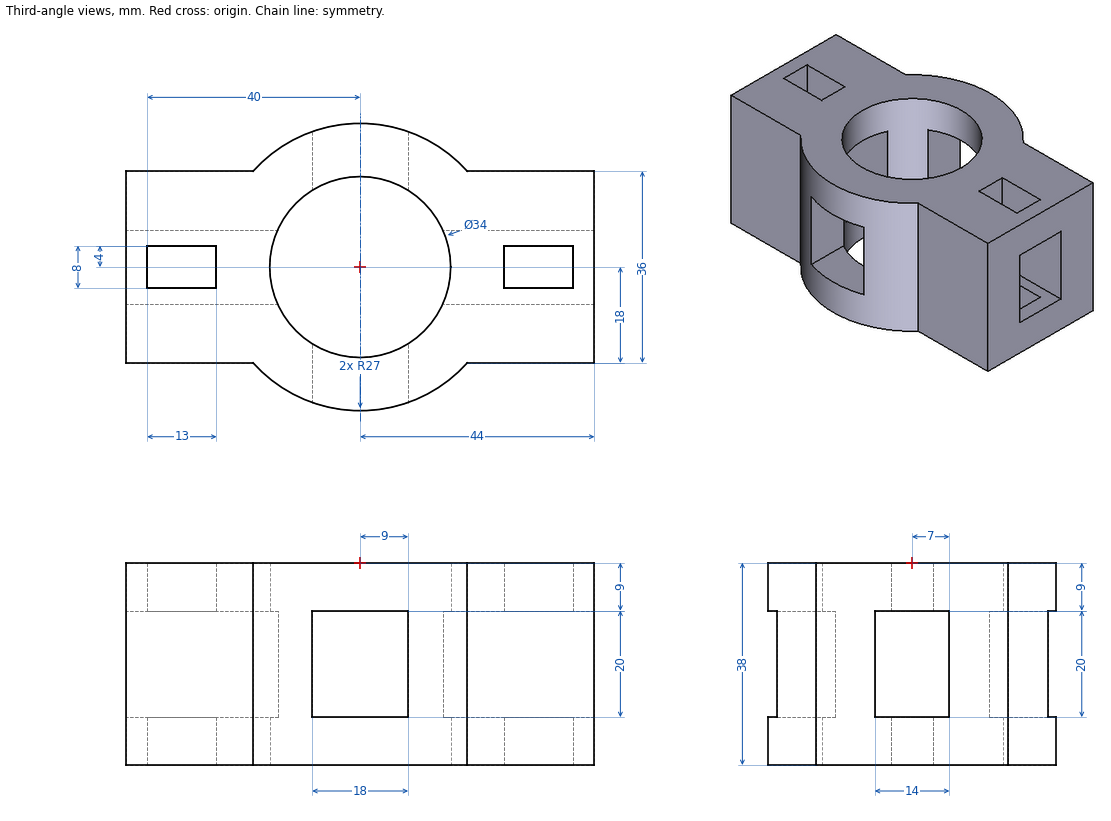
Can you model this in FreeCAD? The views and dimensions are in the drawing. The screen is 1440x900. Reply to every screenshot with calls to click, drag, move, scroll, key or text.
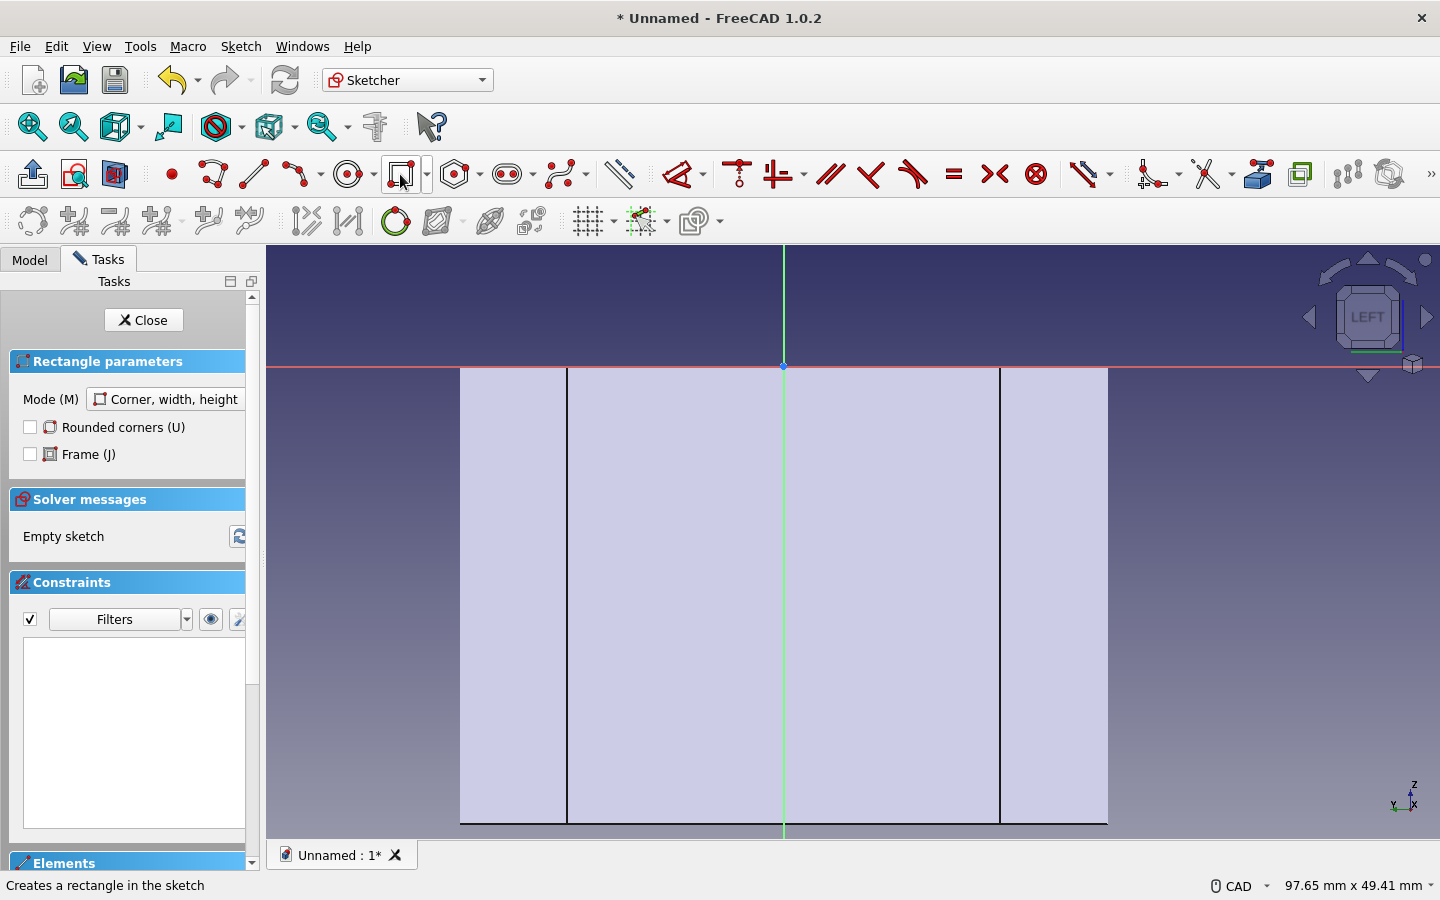
click(700, 475)
click(868, 716)
key(Escape)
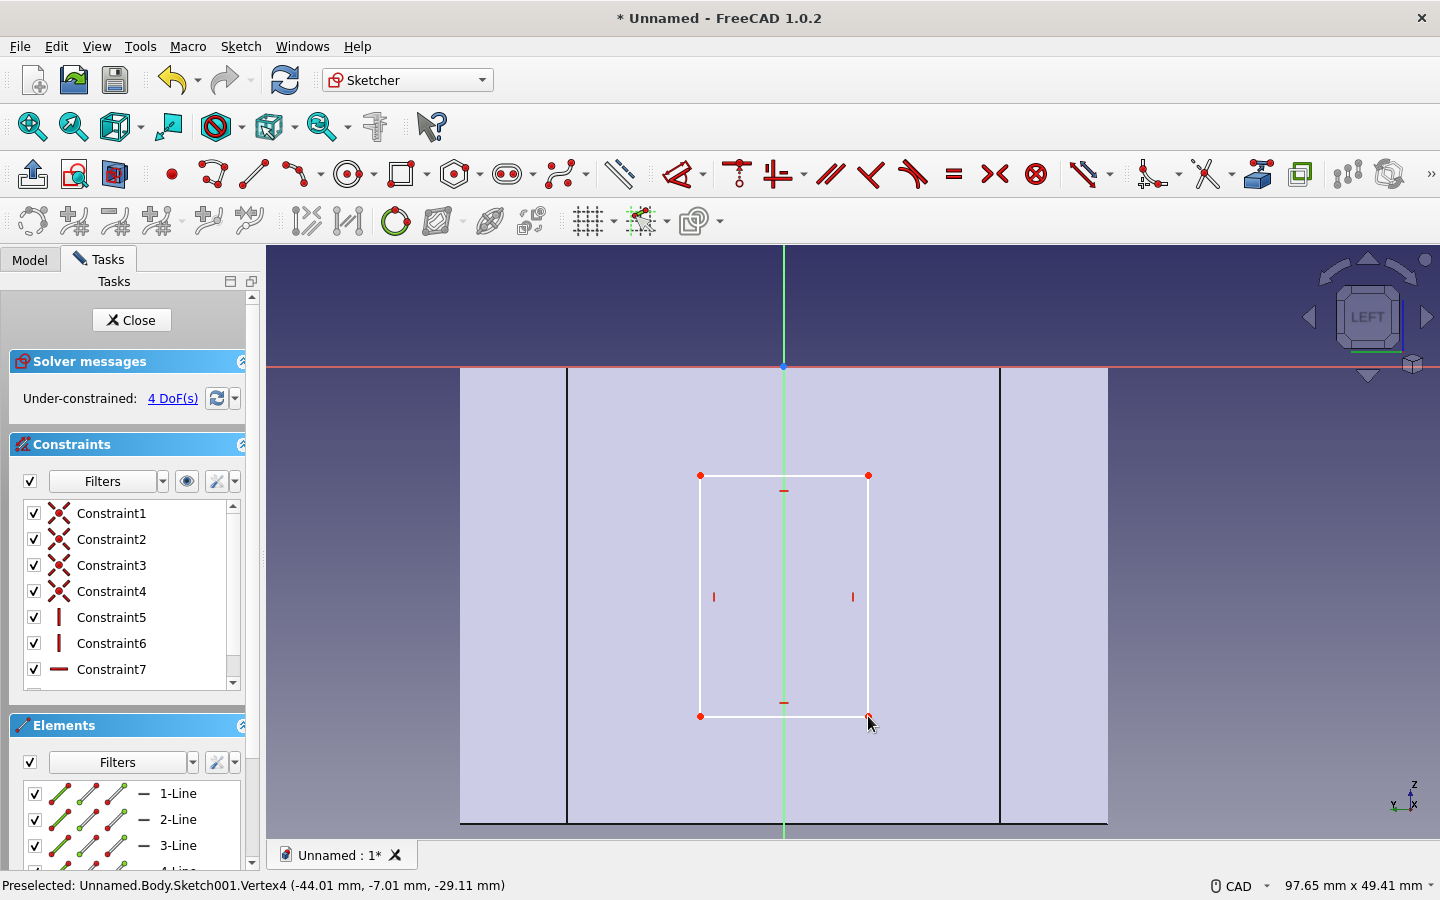
click(676, 174)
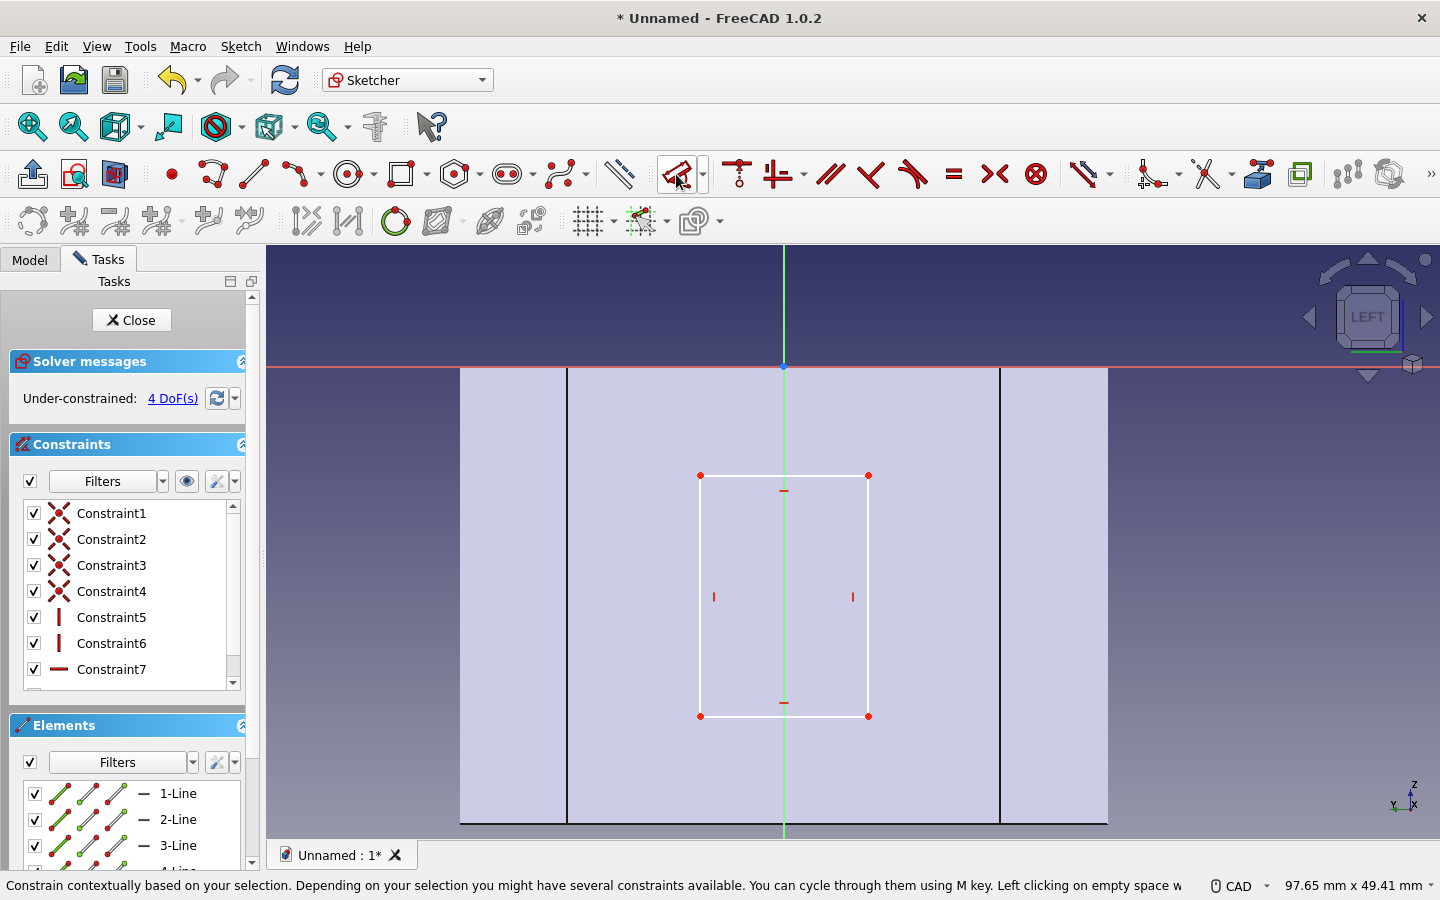
click(700, 548)
click(666, 597)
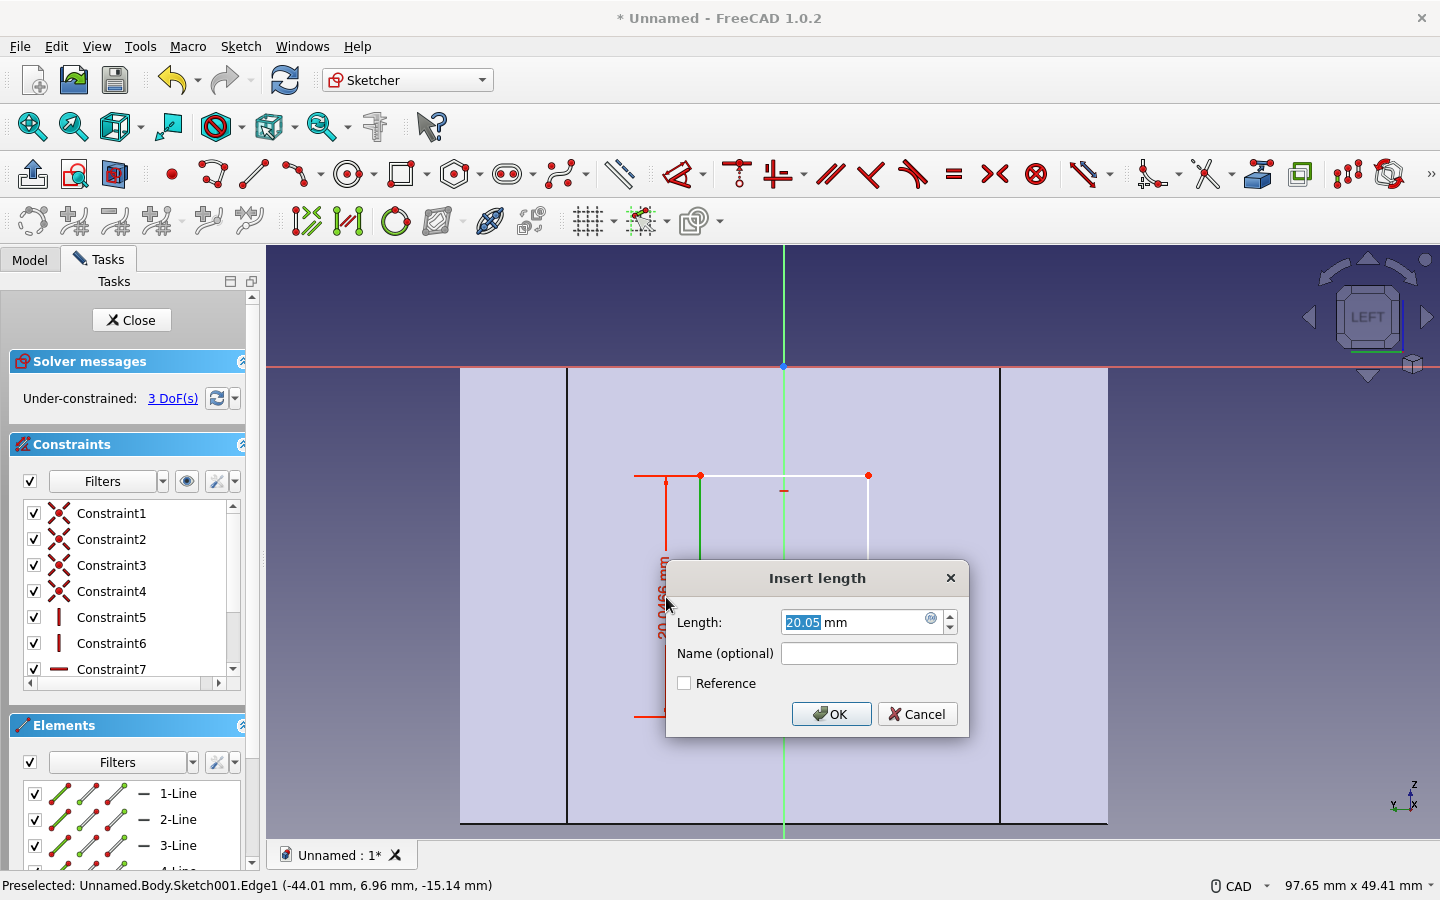
text(20)
key(Return)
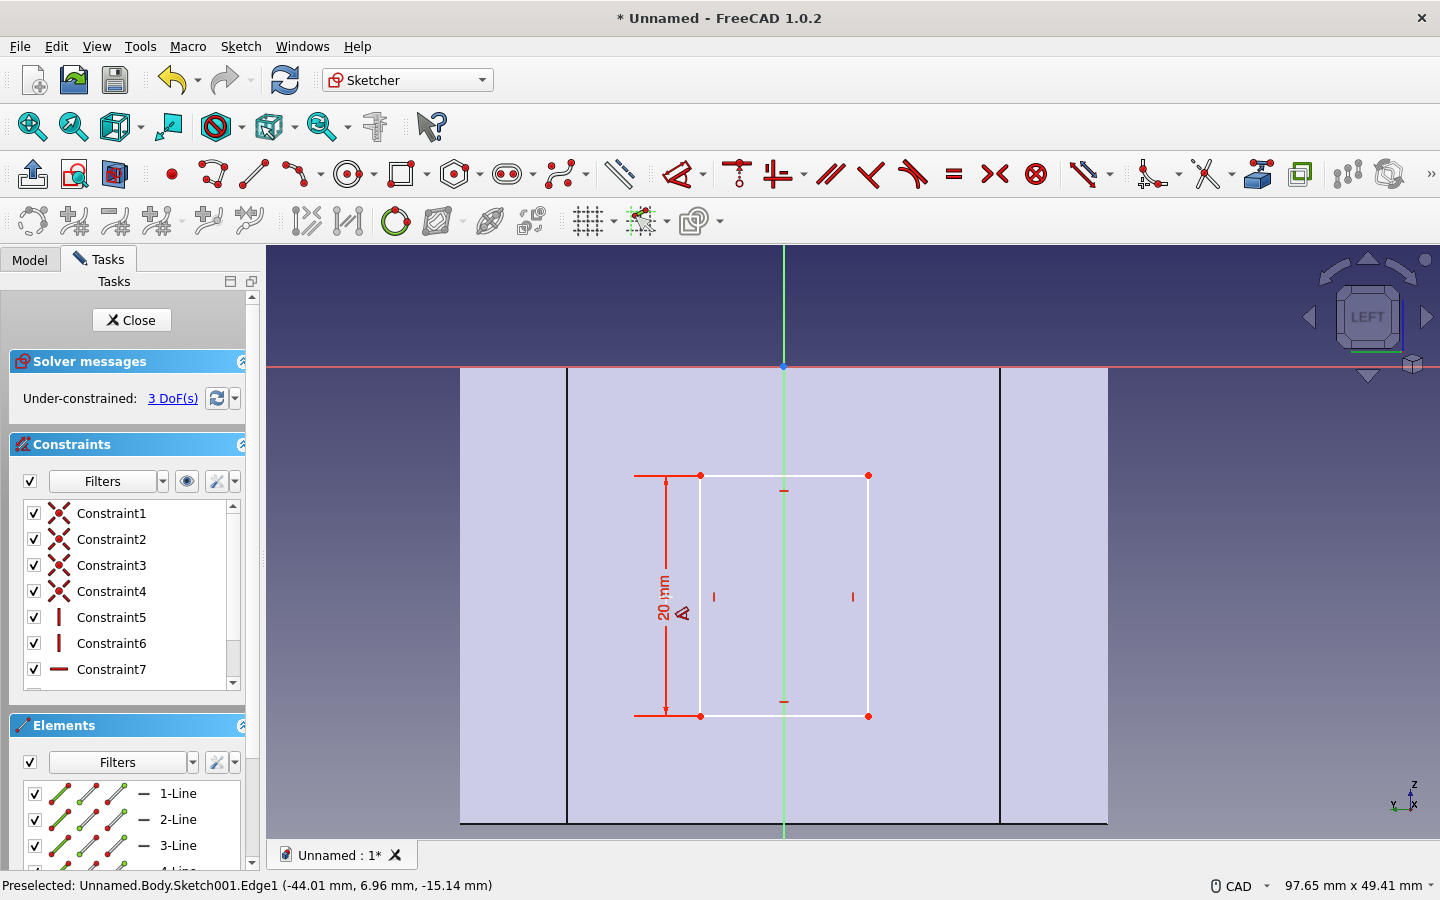
click(750, 716)
click(745, 750)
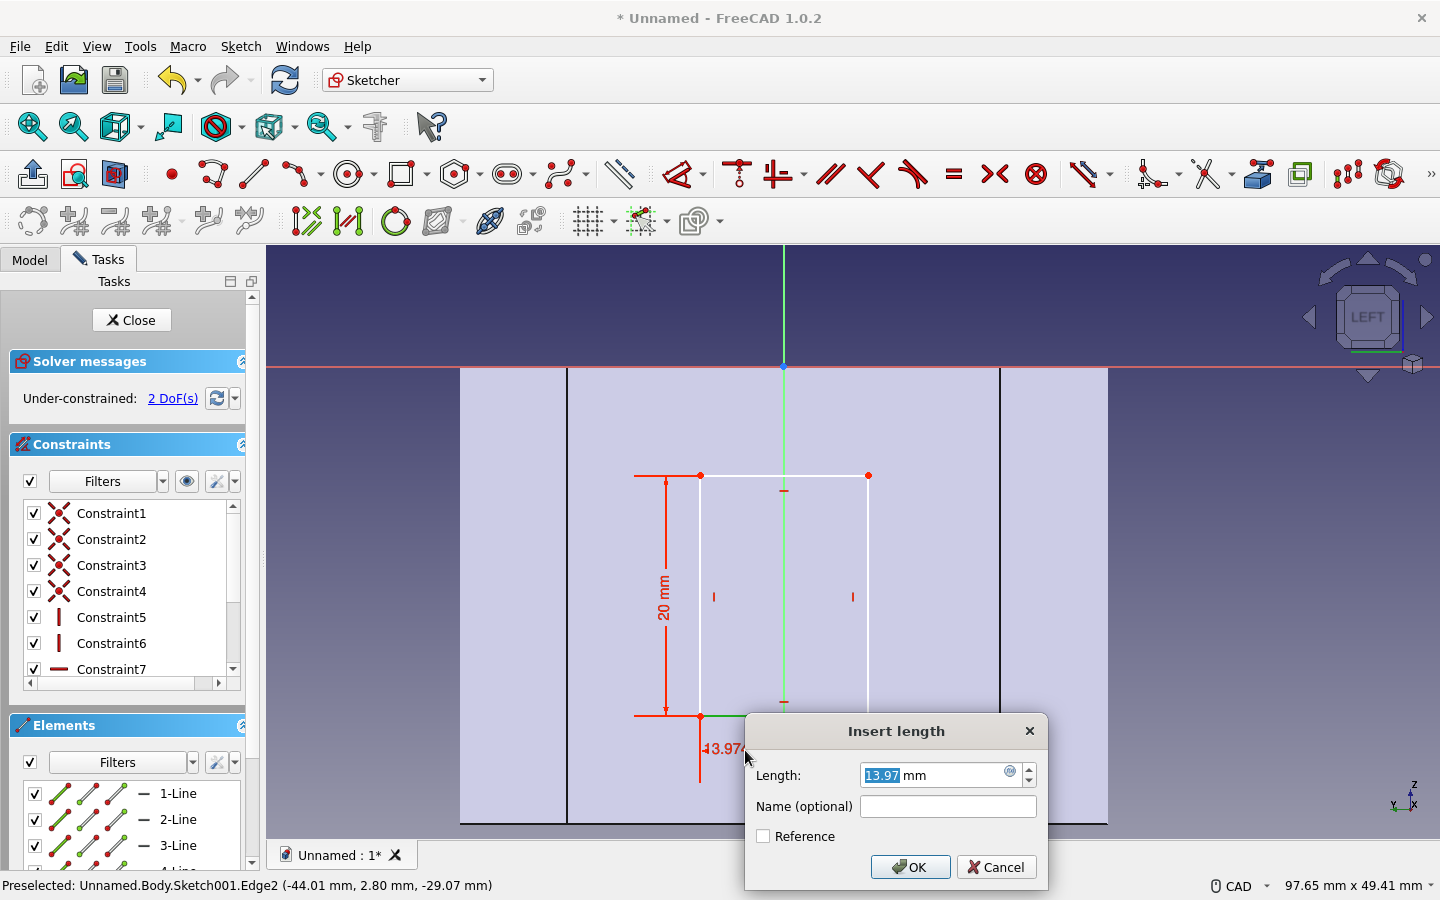
text(14)
key(Return)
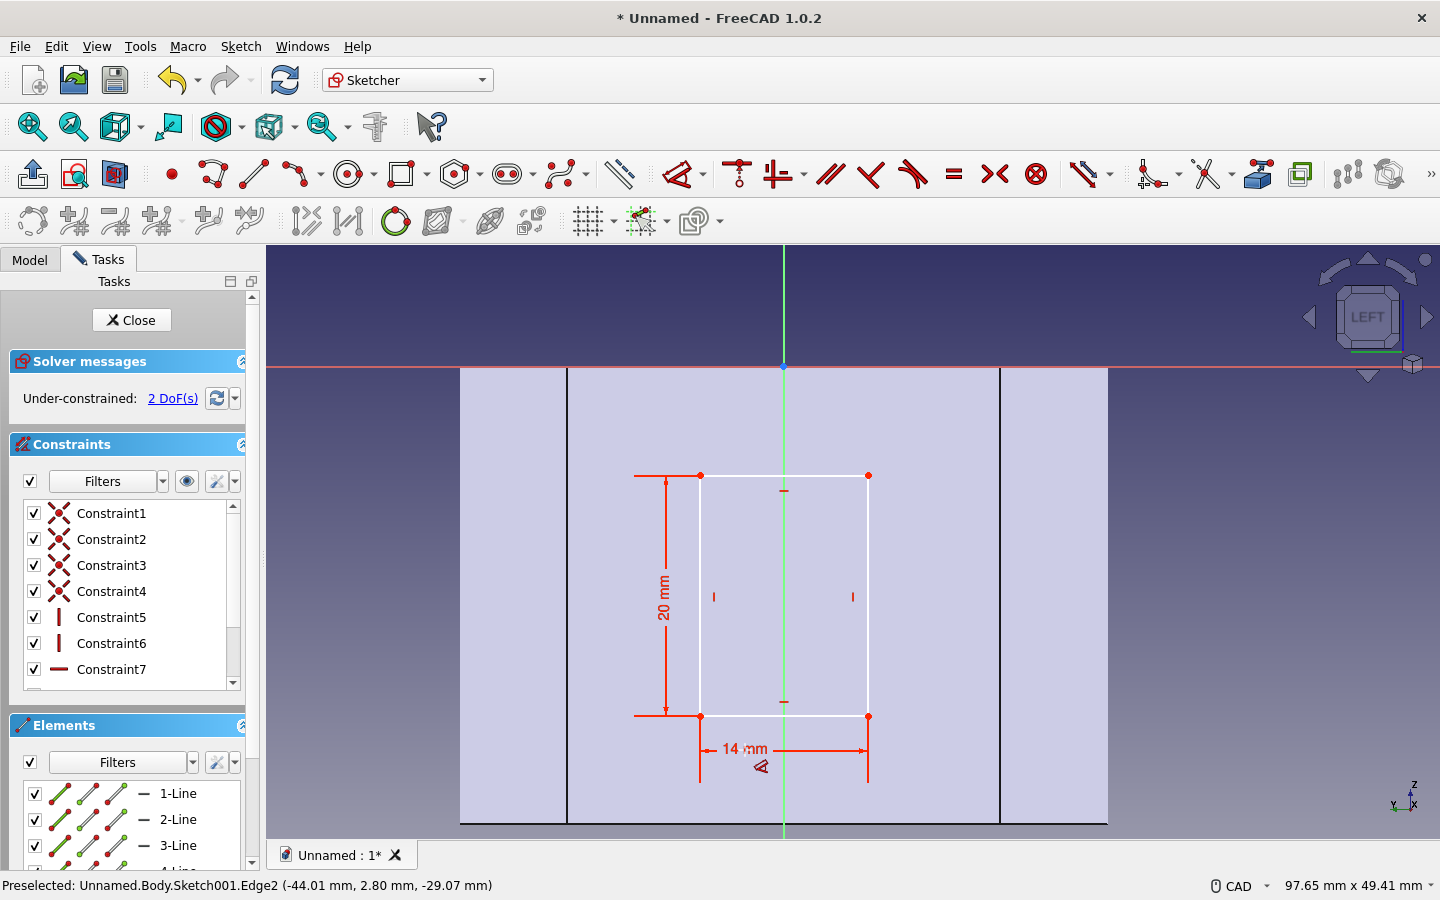
click(700, 476)
click(742, 333)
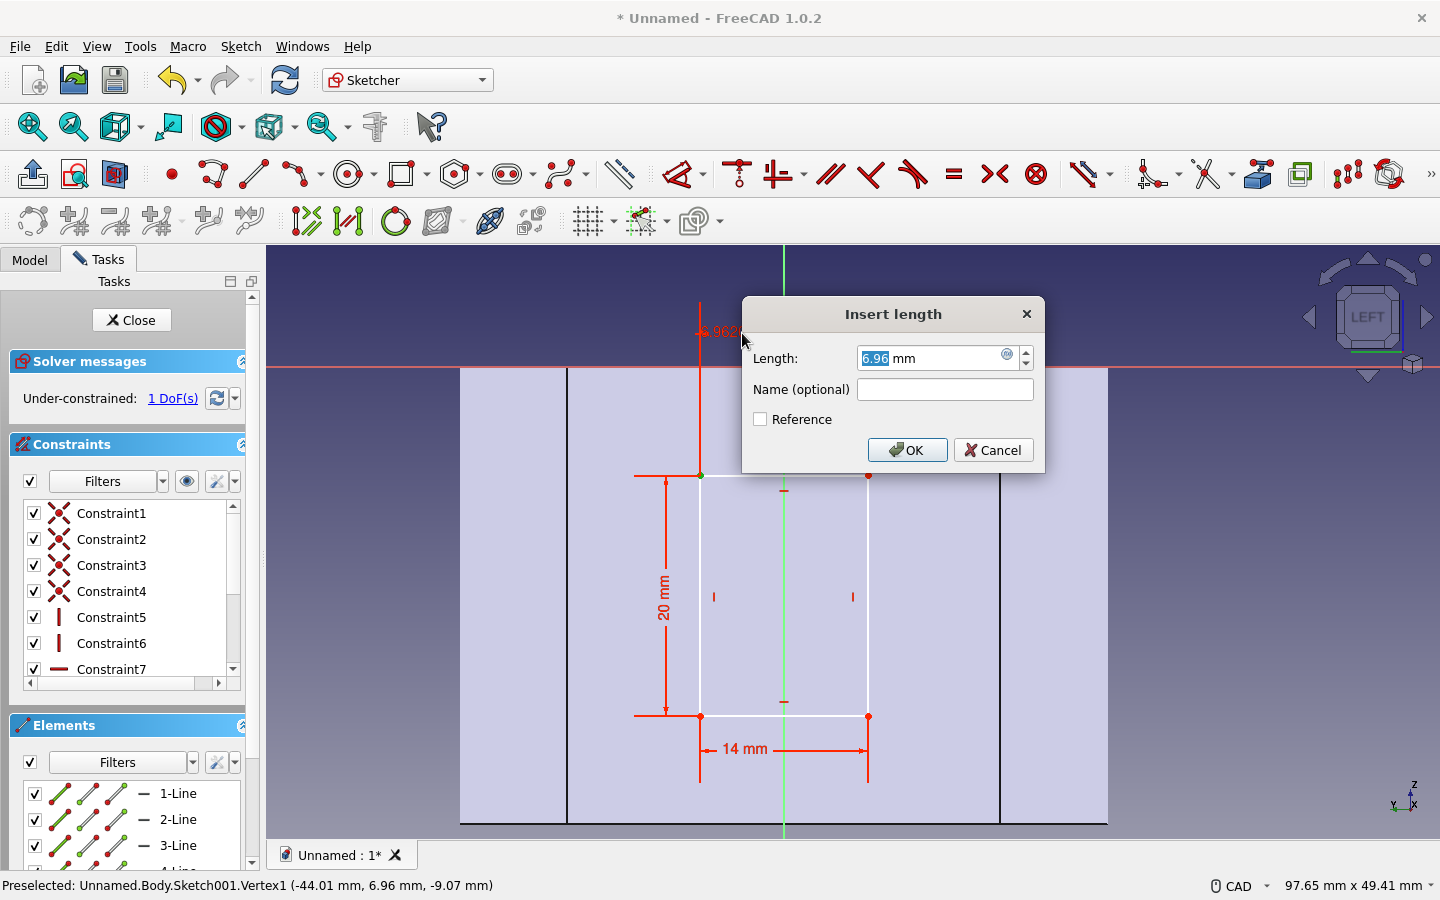
text(7)
key(Return)